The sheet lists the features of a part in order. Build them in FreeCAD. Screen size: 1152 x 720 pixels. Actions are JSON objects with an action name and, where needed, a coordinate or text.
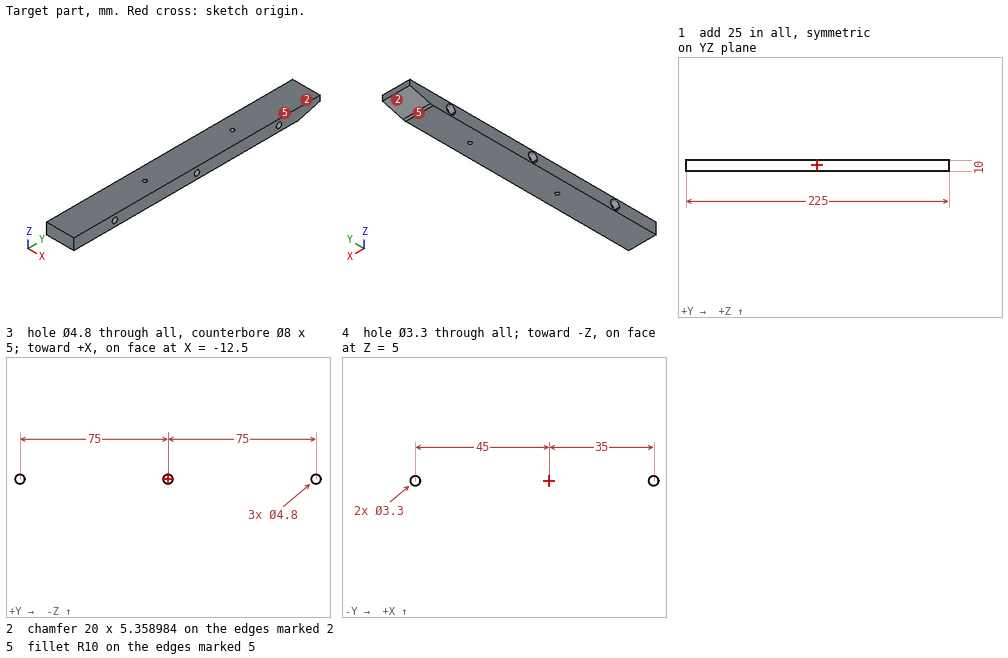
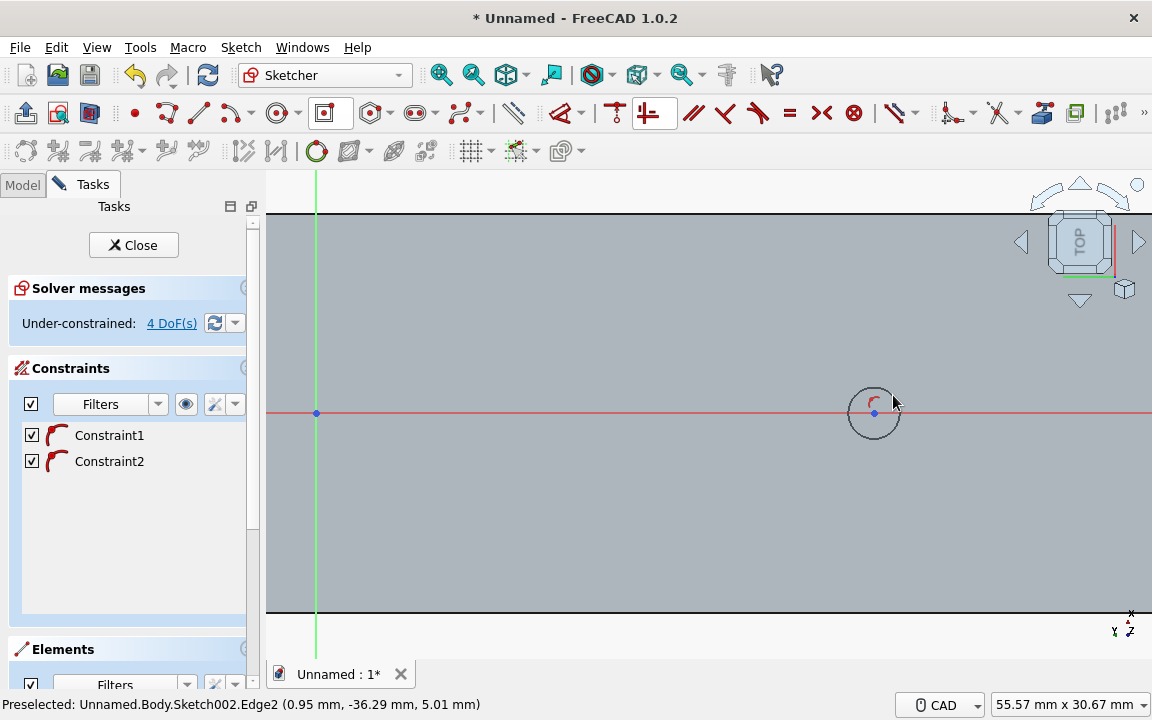
{"action": "scroll", "coordinate": [876, 415], "scroll_direction": "down", "scroll_amount": 5}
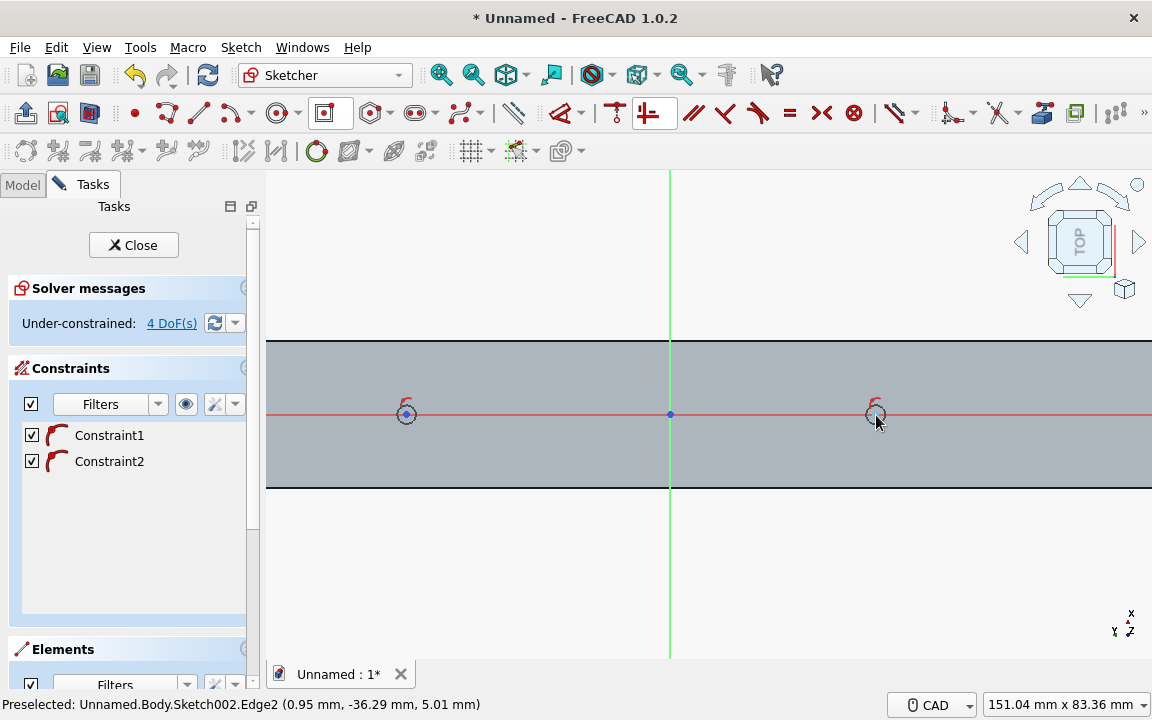
{"action": "scroll", "coordinate": [413, 408], "scroll_direction": "up", "scroll_amount": 4}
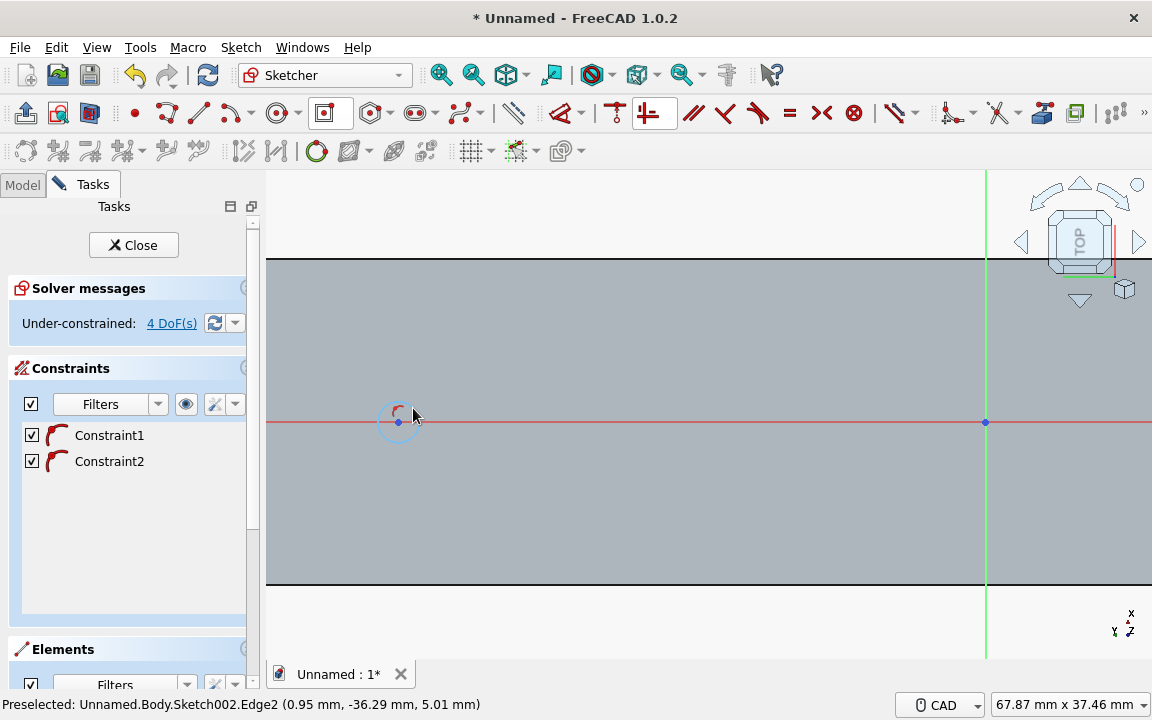
{"action": "left_click", "coordinate": [413, 408]}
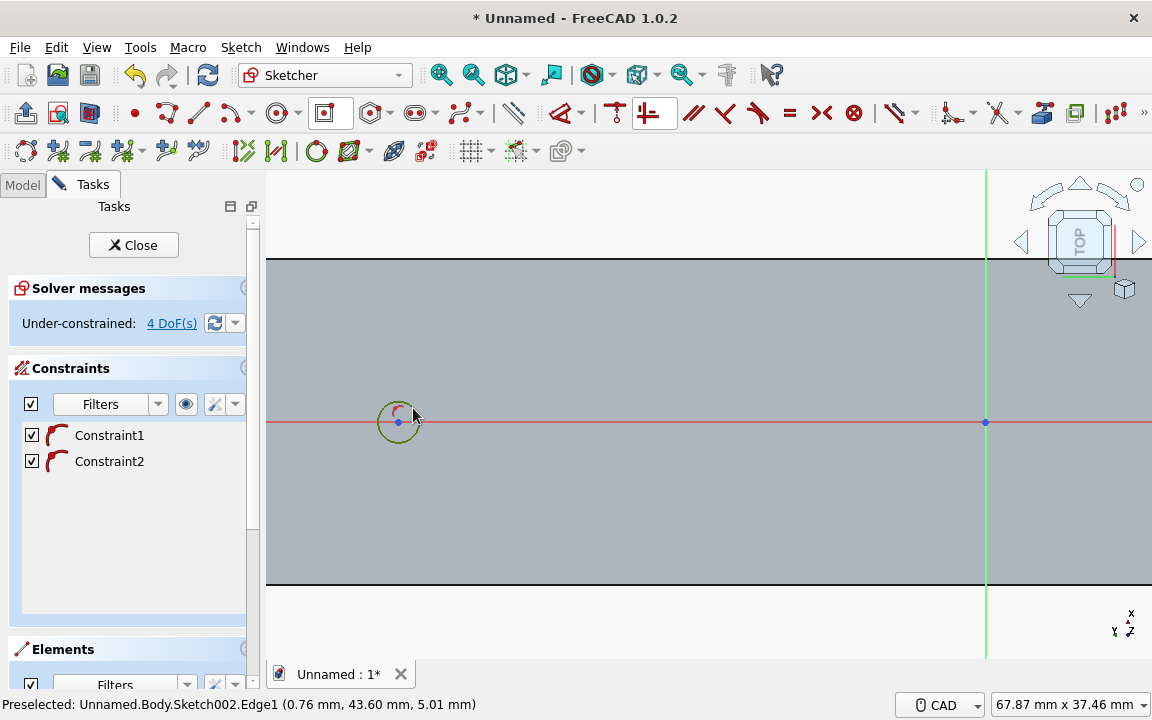
{"action": "scroll", "coordinate": [412, 408], "scroll_direction": "down", "scroll_amount": 4}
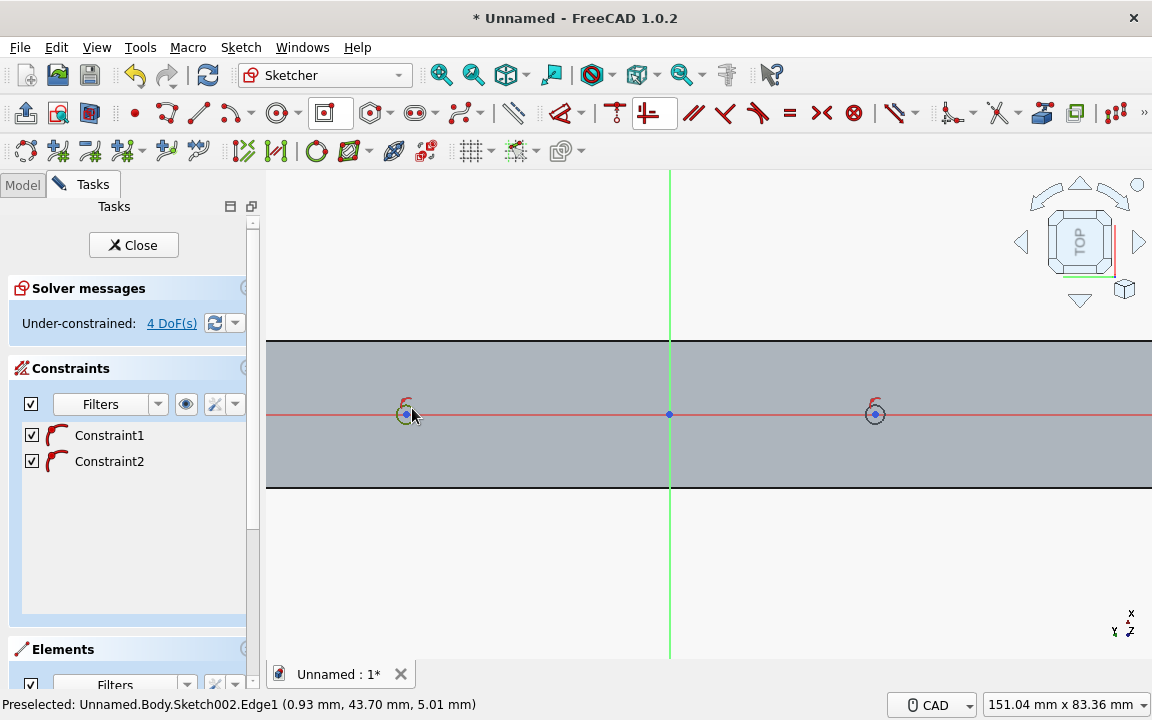
{"action": "scroll", "coordinate": [882, 408], "scroll_direction": "up", "scroll_amount": 4}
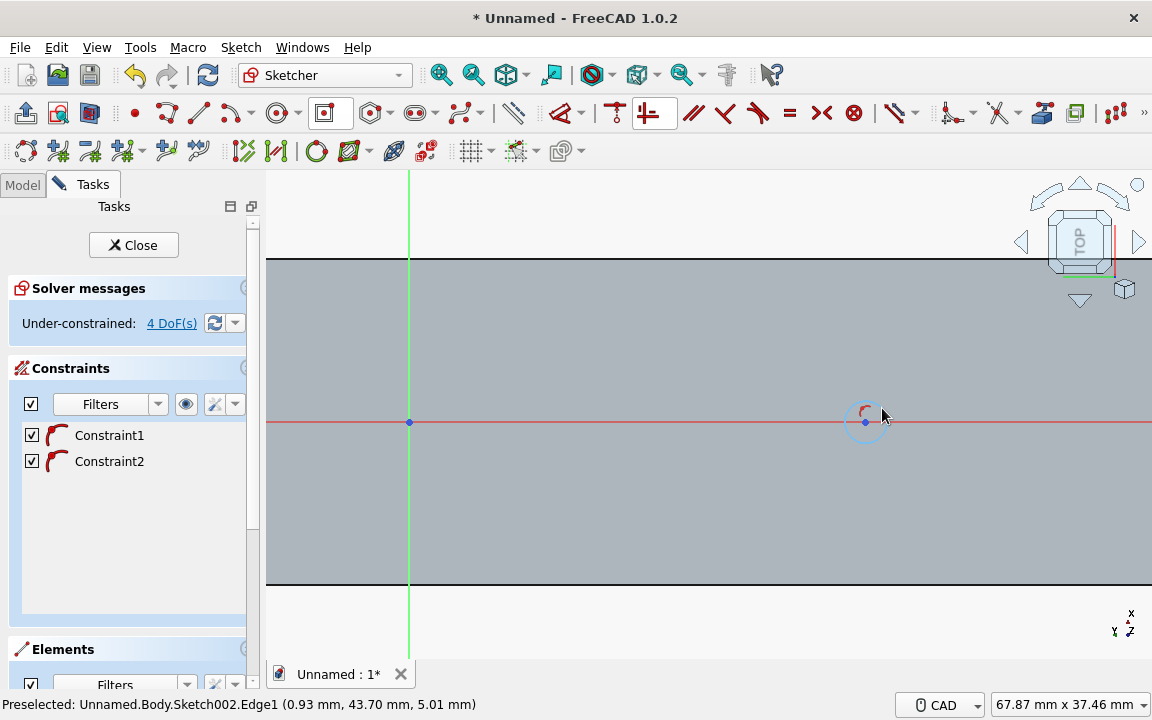
{"action": "left_click", "coordinate": [881, 407]}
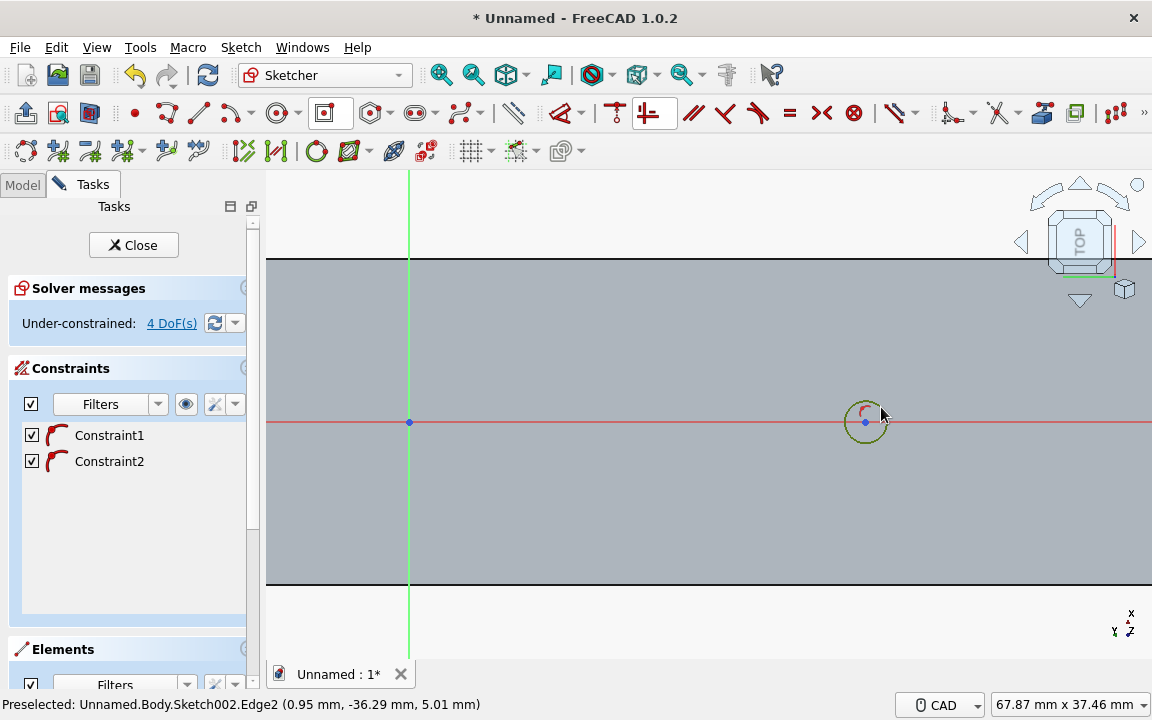
{"action": "left_click", "coordinate": [790, 114]}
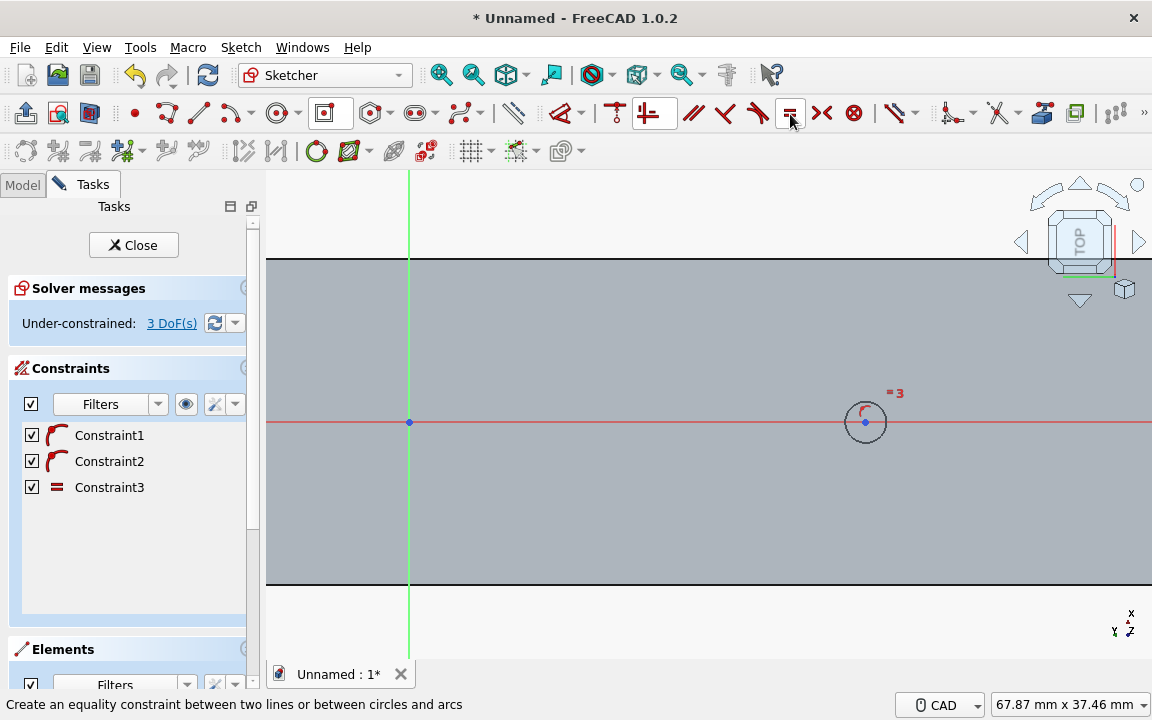
{"action": "left_click", "coordinate": [560, 114]}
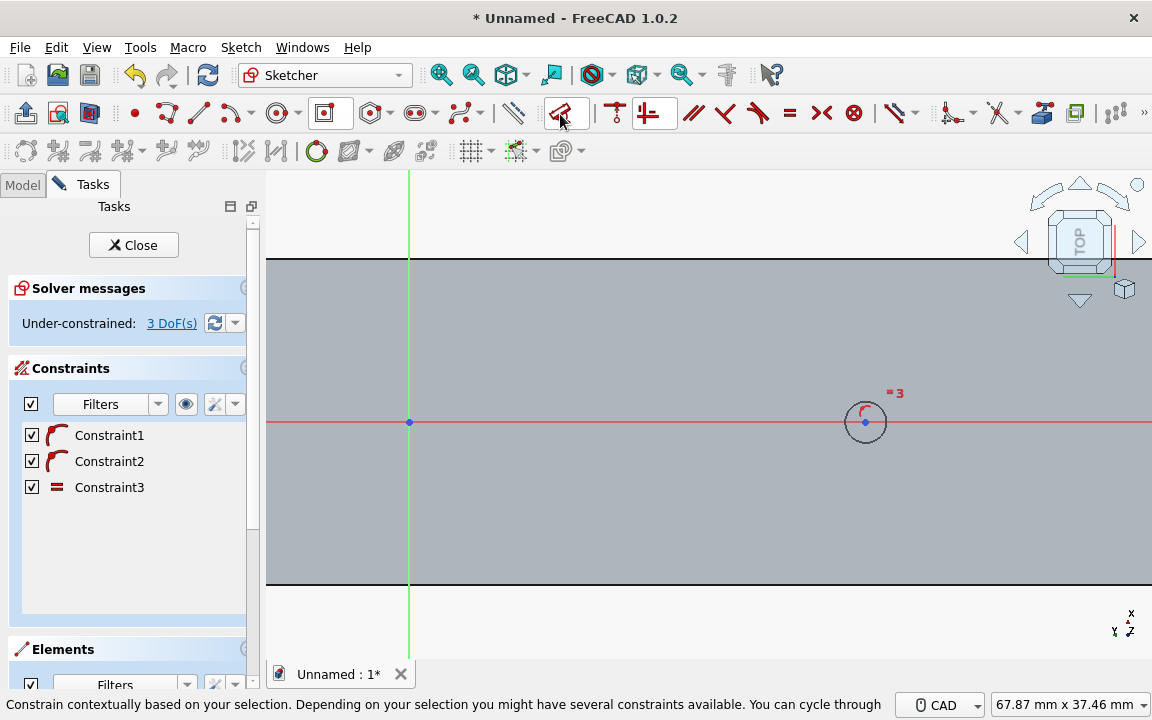
{"action": "scroll", "coordinate": [883, 408], "scroll_direction": "down", "scroll_amount": 4}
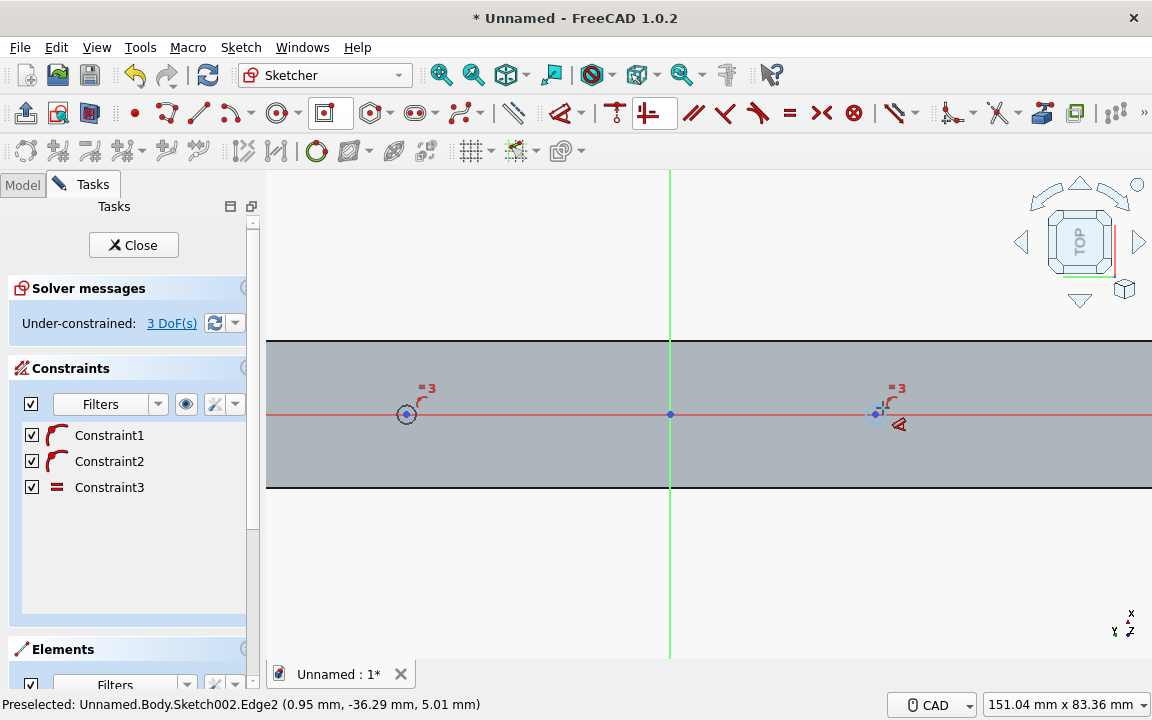
{"action": "scroll", "coordinate": [413, 408], "scroll_direction": "up", "scroll_amount": 4}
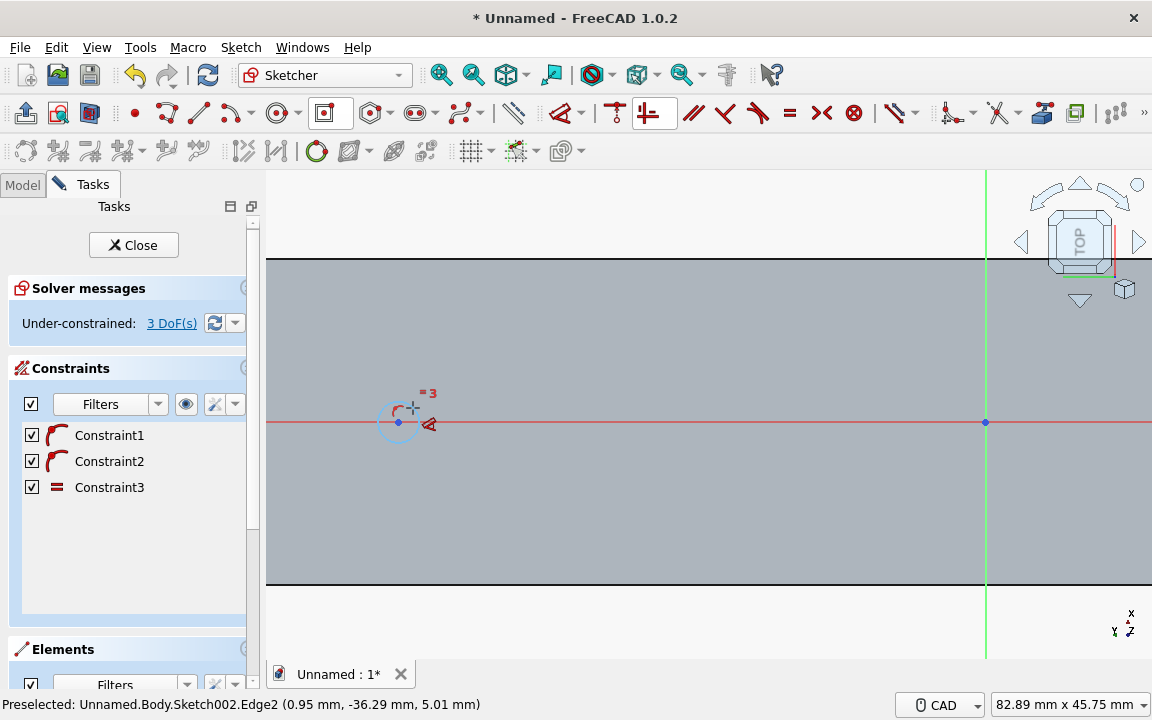
{"action": "left_click", "coordinate": [413, 408]}
{"action": "left_click", "coordinate": [436, 385]}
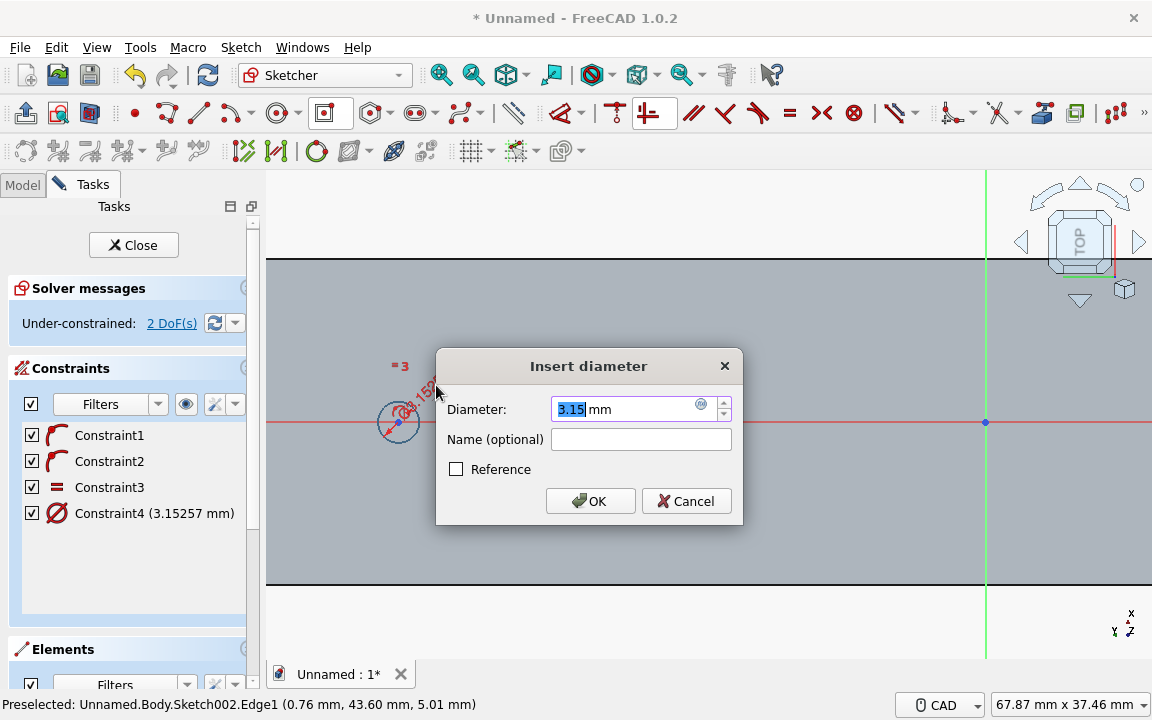
{"action": "type", "text": "3.3"}
{"action": "key", "text": "Return"}